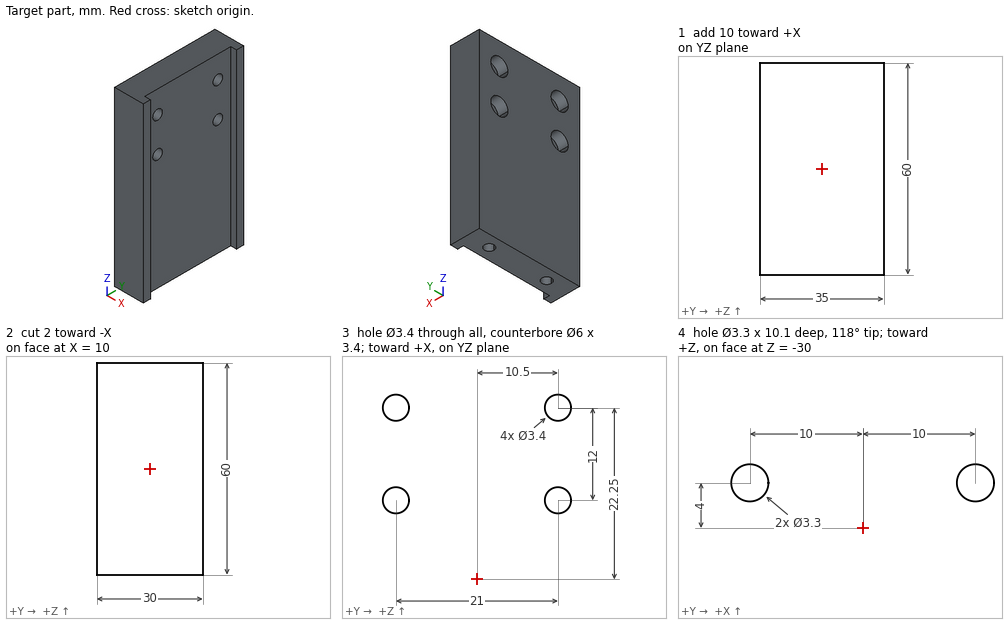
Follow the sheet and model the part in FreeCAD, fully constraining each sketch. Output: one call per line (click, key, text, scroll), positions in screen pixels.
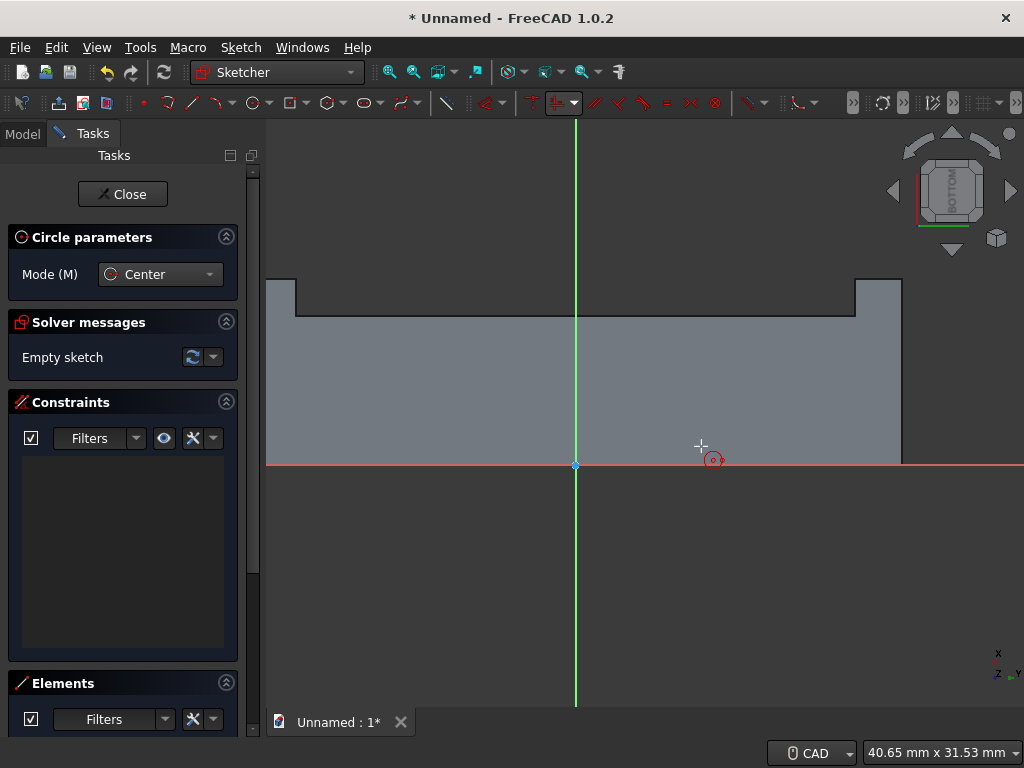
click(389, 391)
move(411, 369)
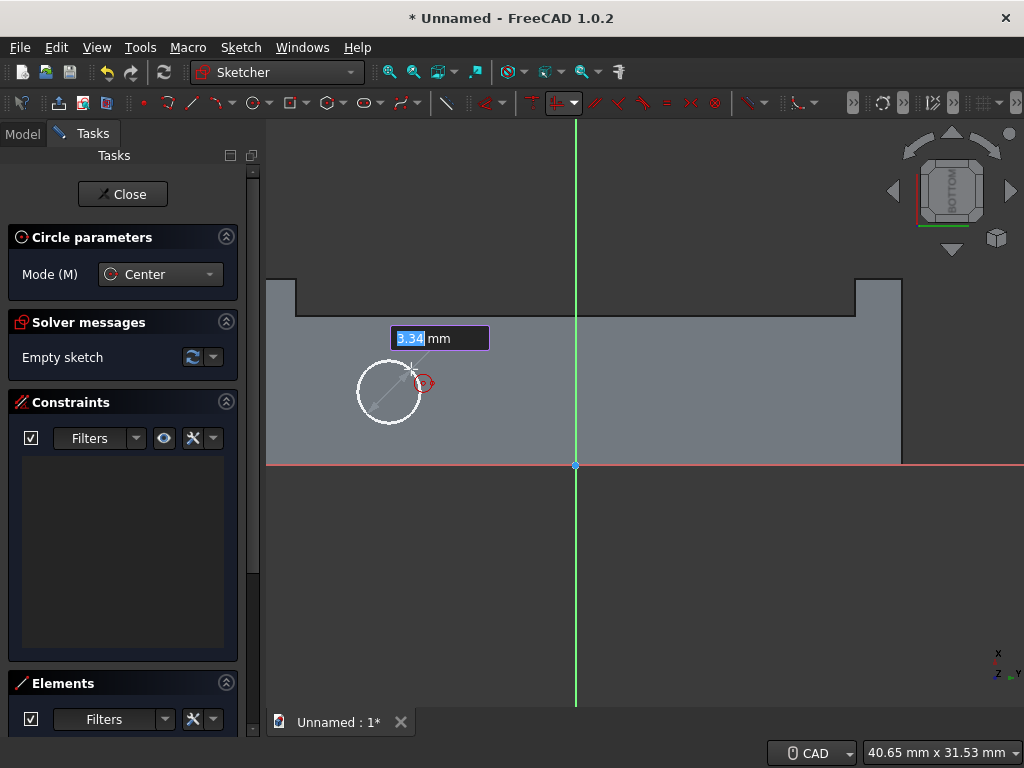
text(3.3)
key(Return)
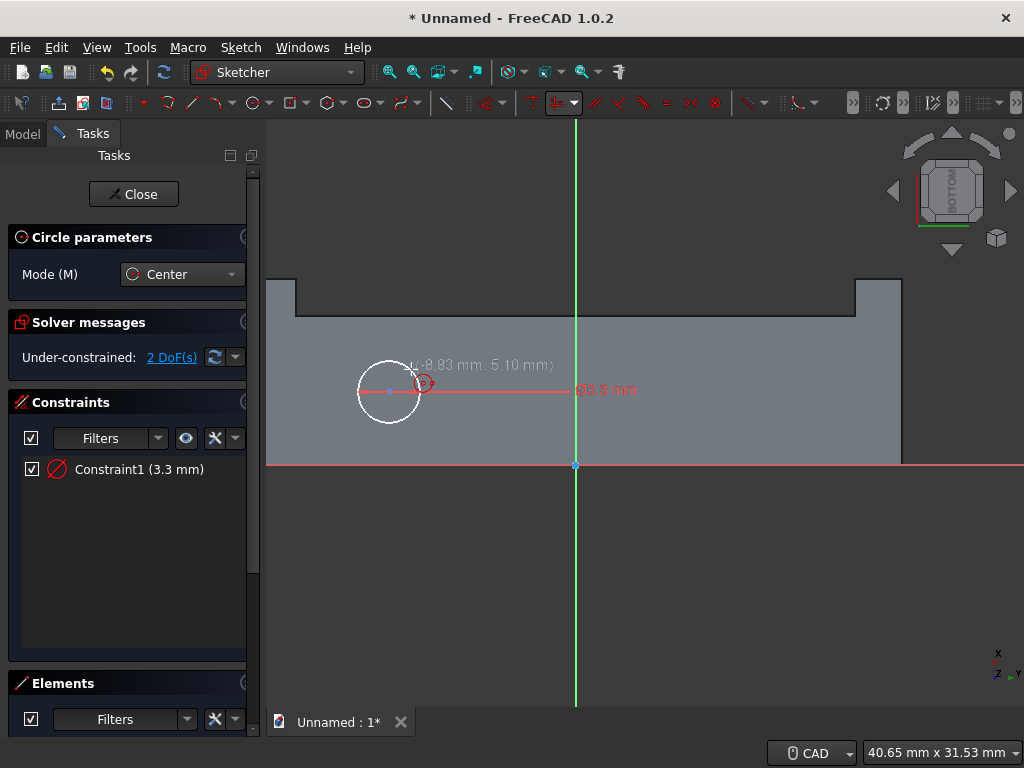
click(762, 391)
move(784, 369)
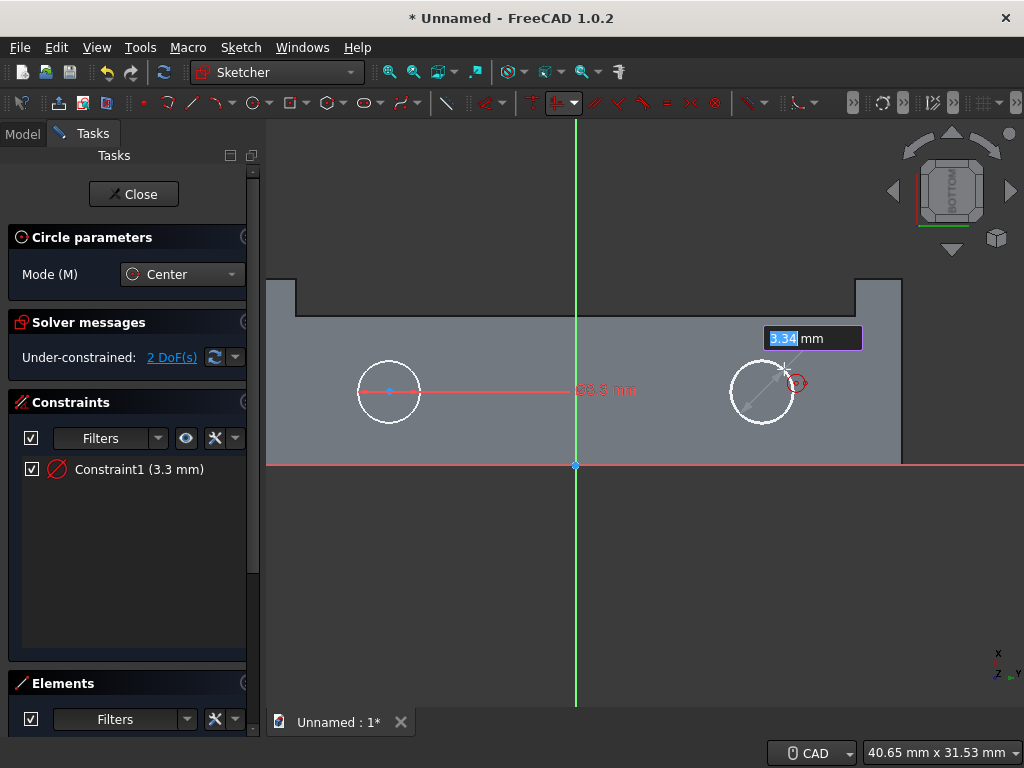
text(3.3)
key(Return)
key(Escape)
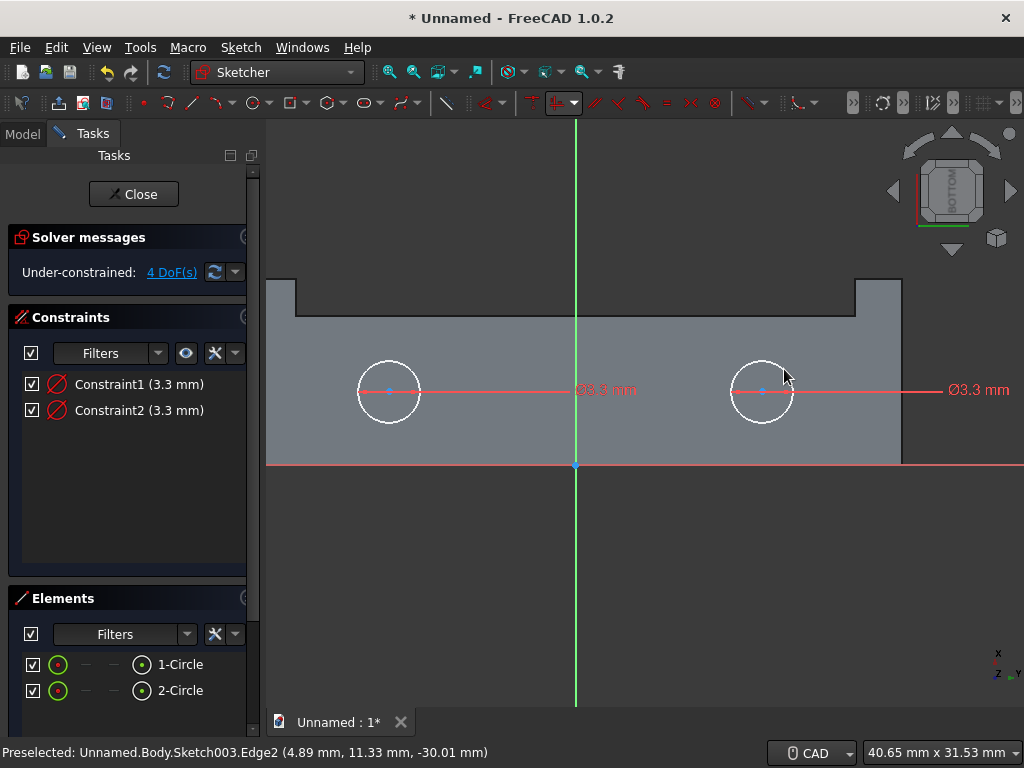
click(389, 392)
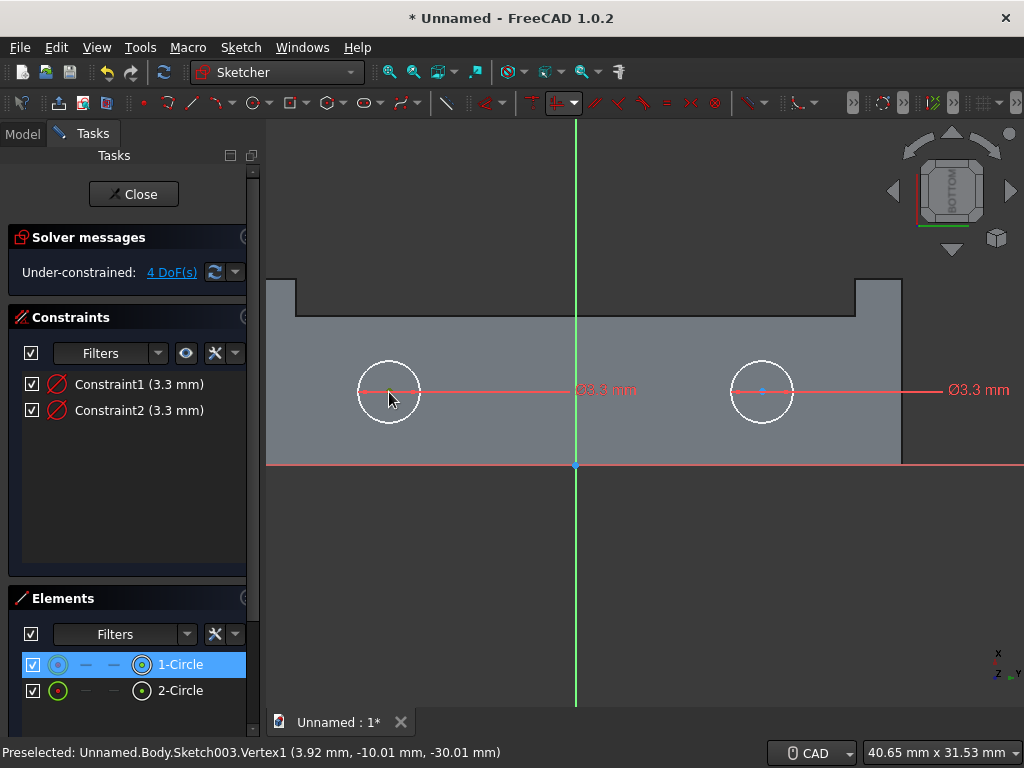
click(762, 392)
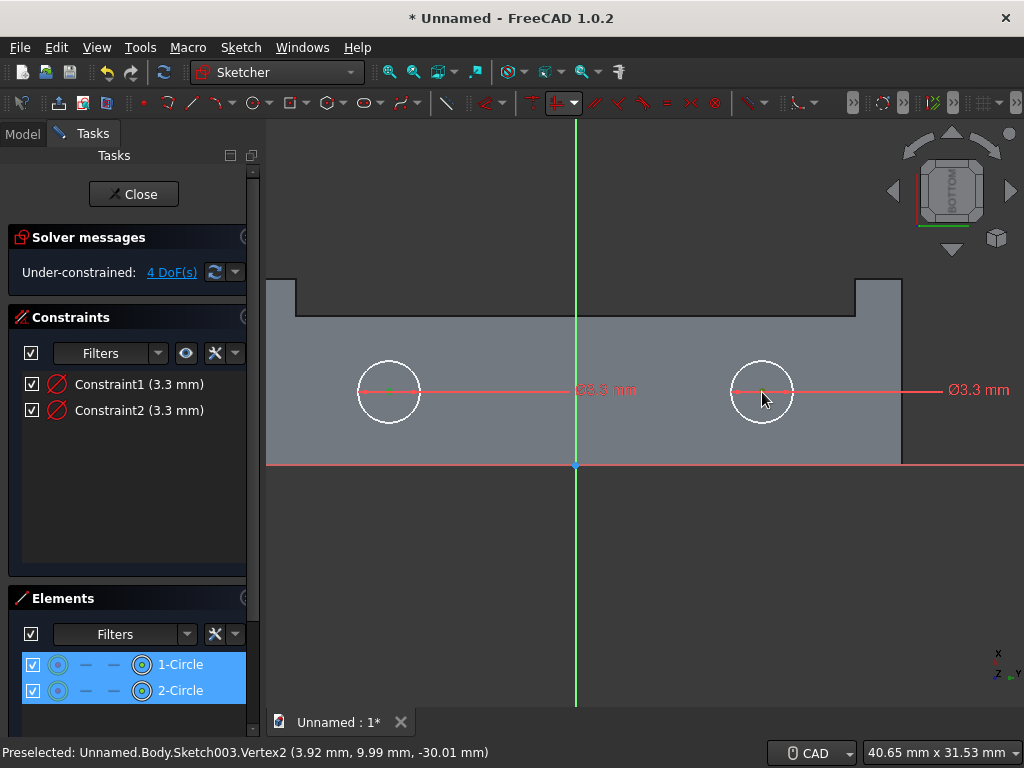
click(576, 104)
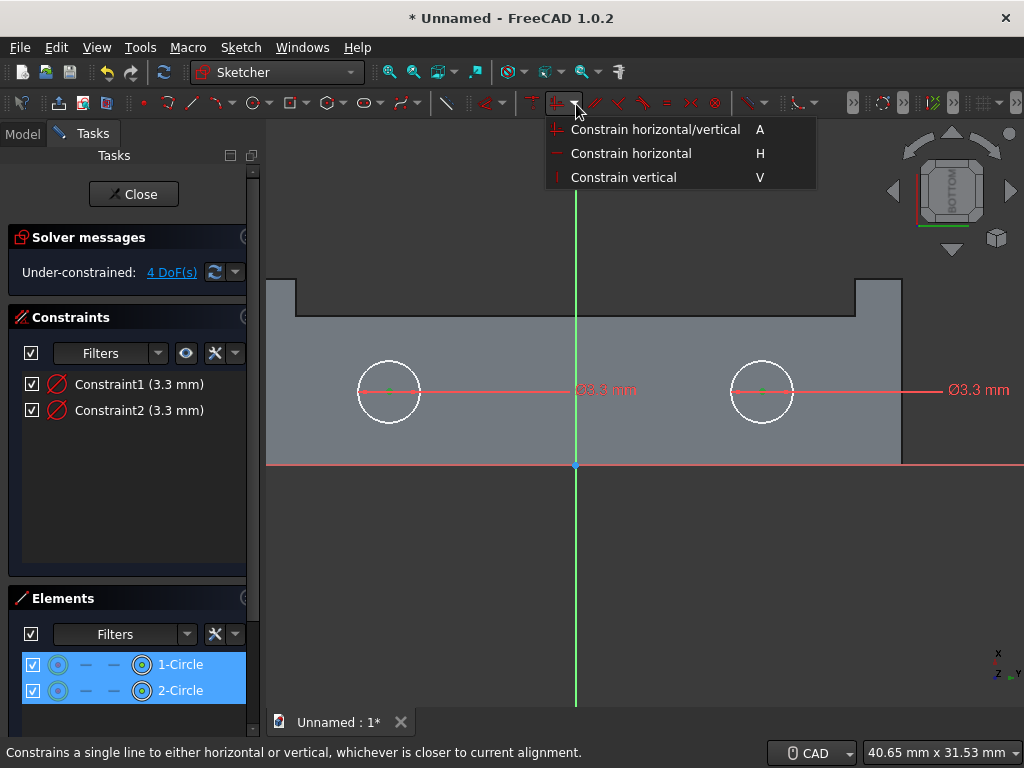
click(681, 153)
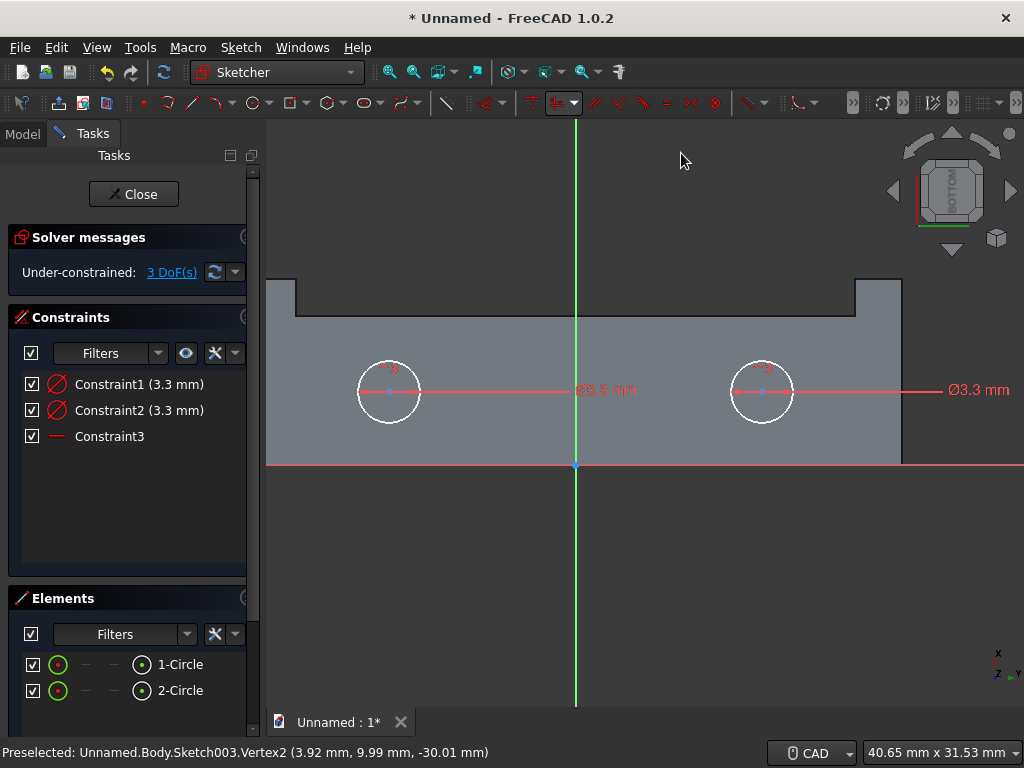
click(486, 104)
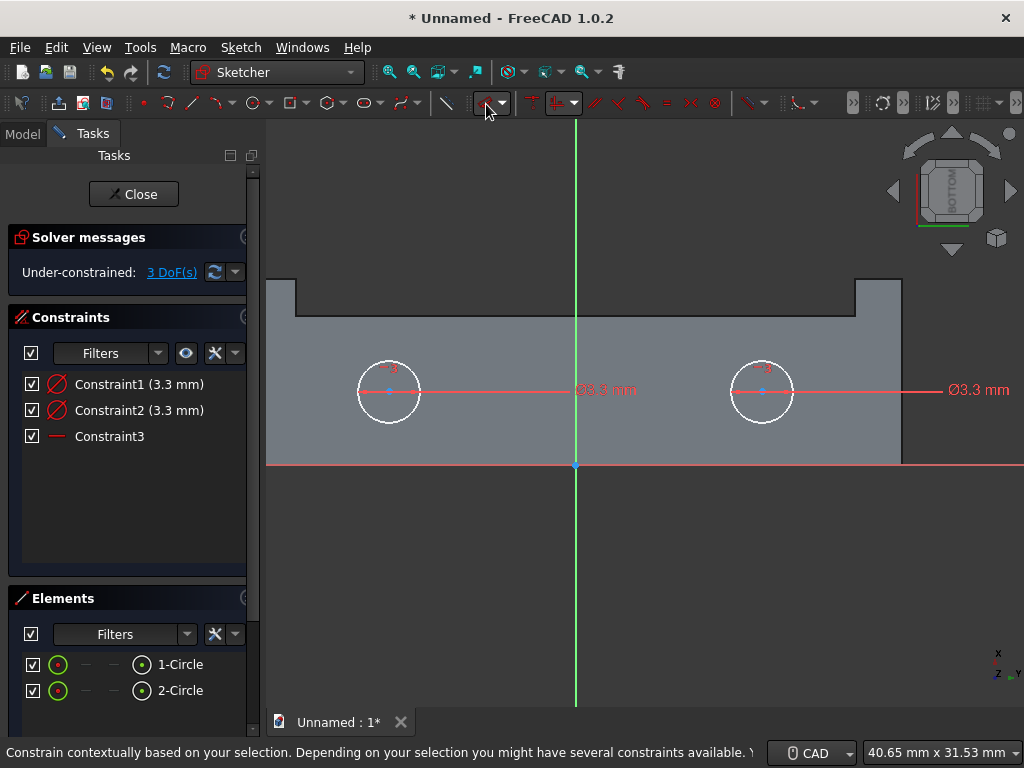
click(389, 392)
click(355, 429)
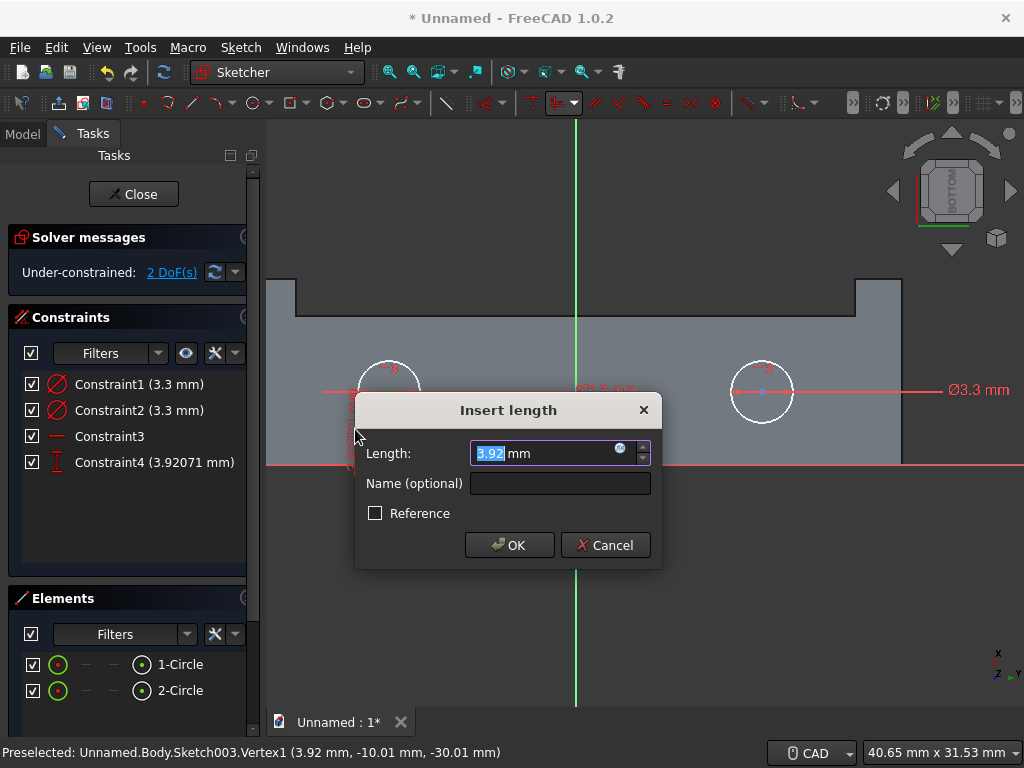
text(4)
key(Return)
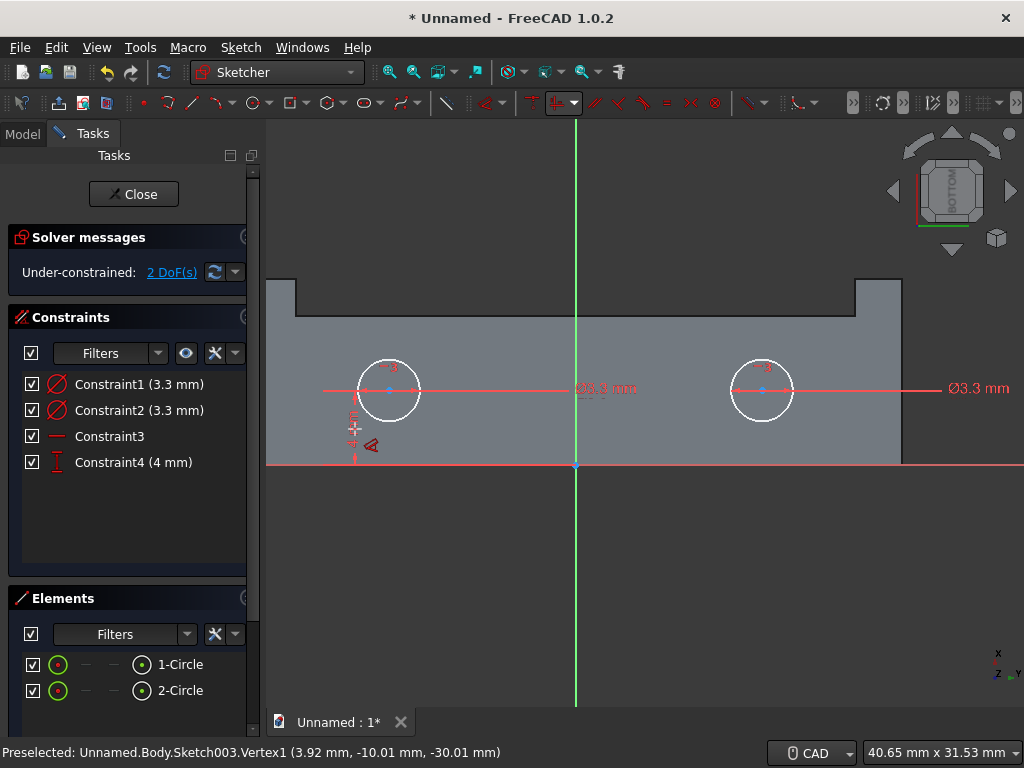
click(389, 391)
click(482, 499)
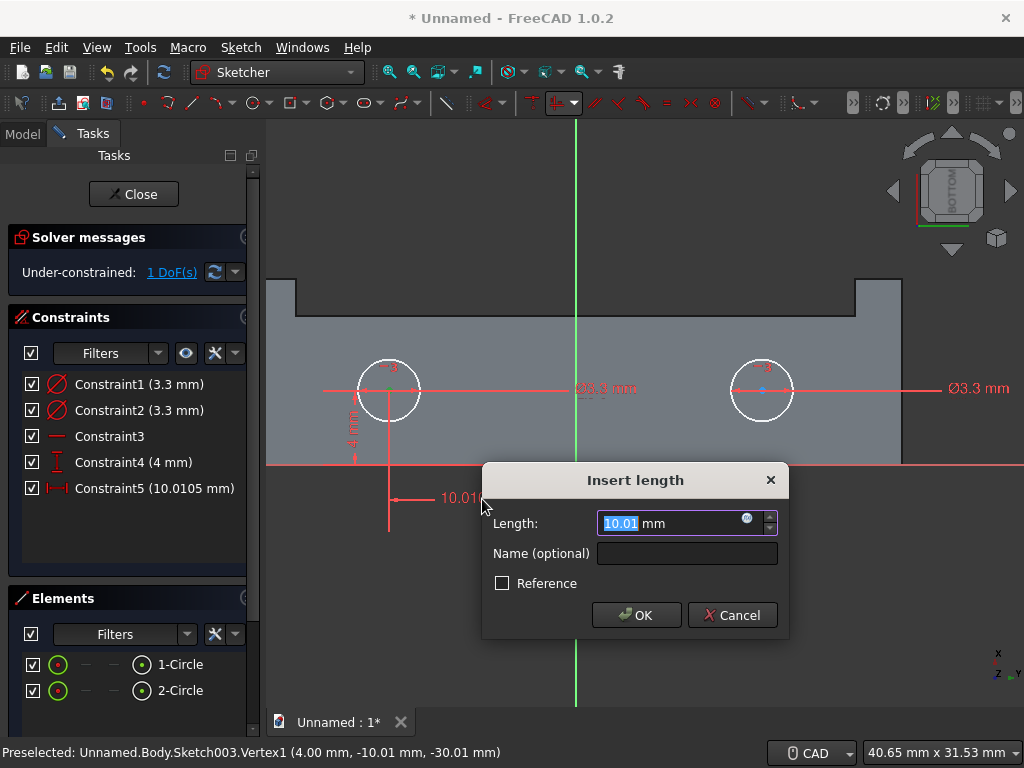
text(10)
key(Return)